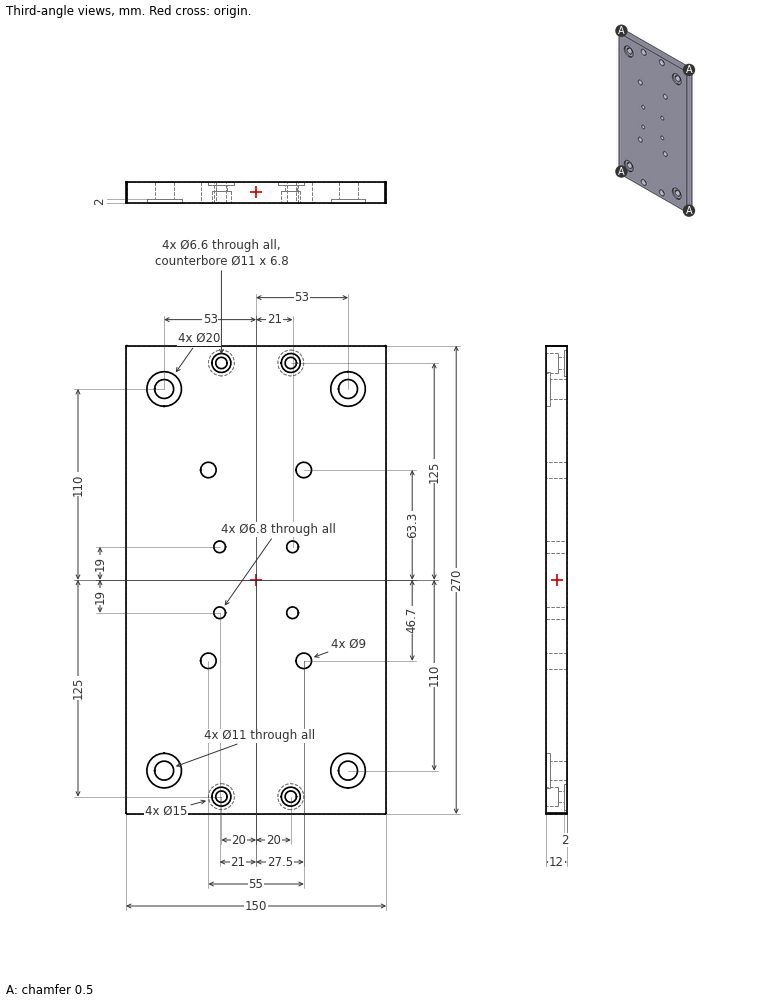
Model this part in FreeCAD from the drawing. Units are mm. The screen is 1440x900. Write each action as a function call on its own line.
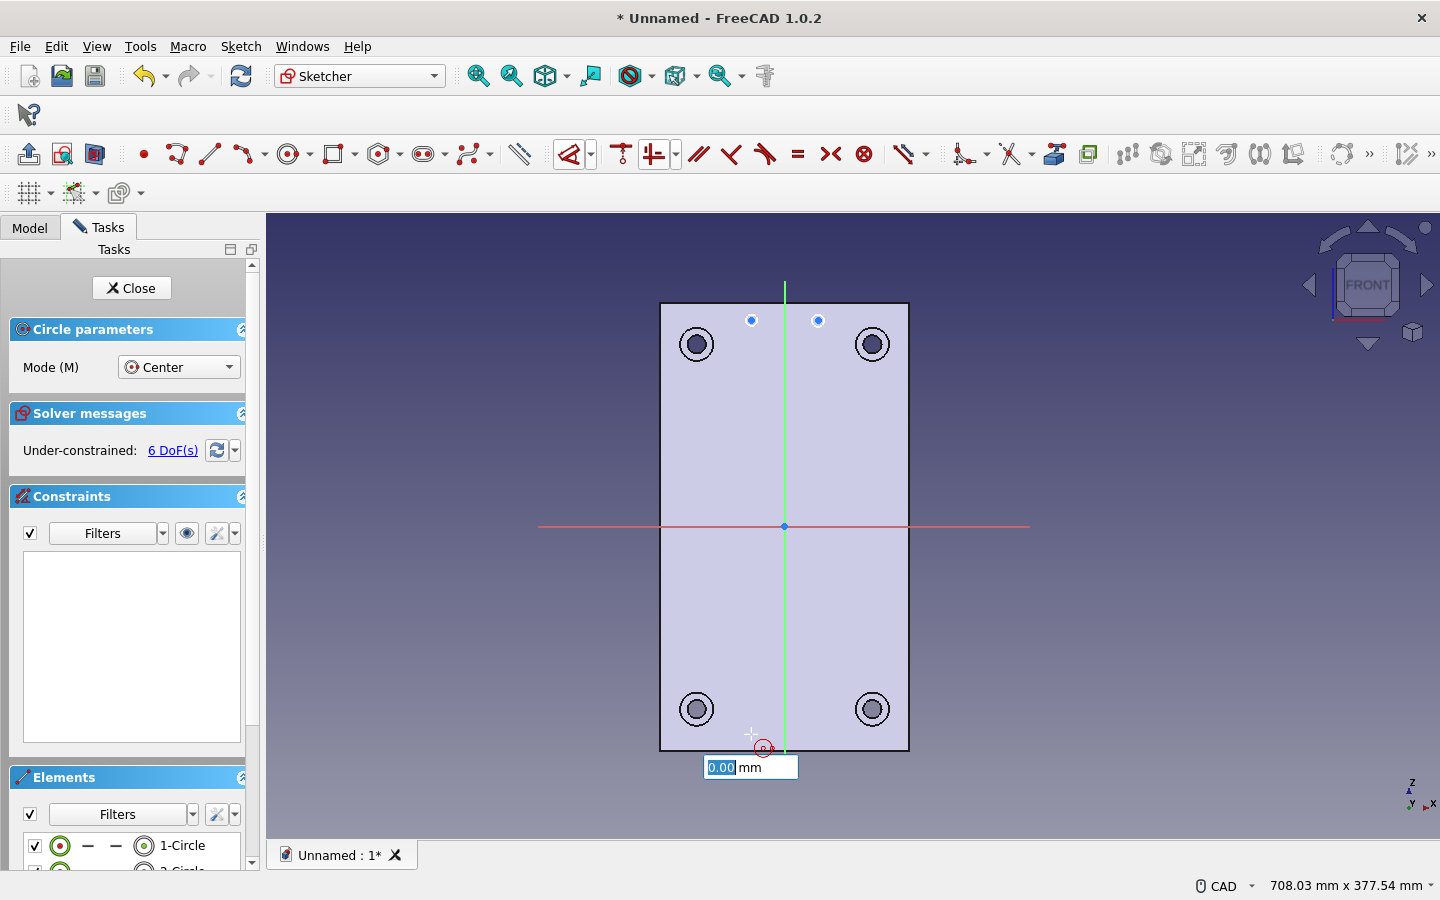
scroll(755, 730, up, 6)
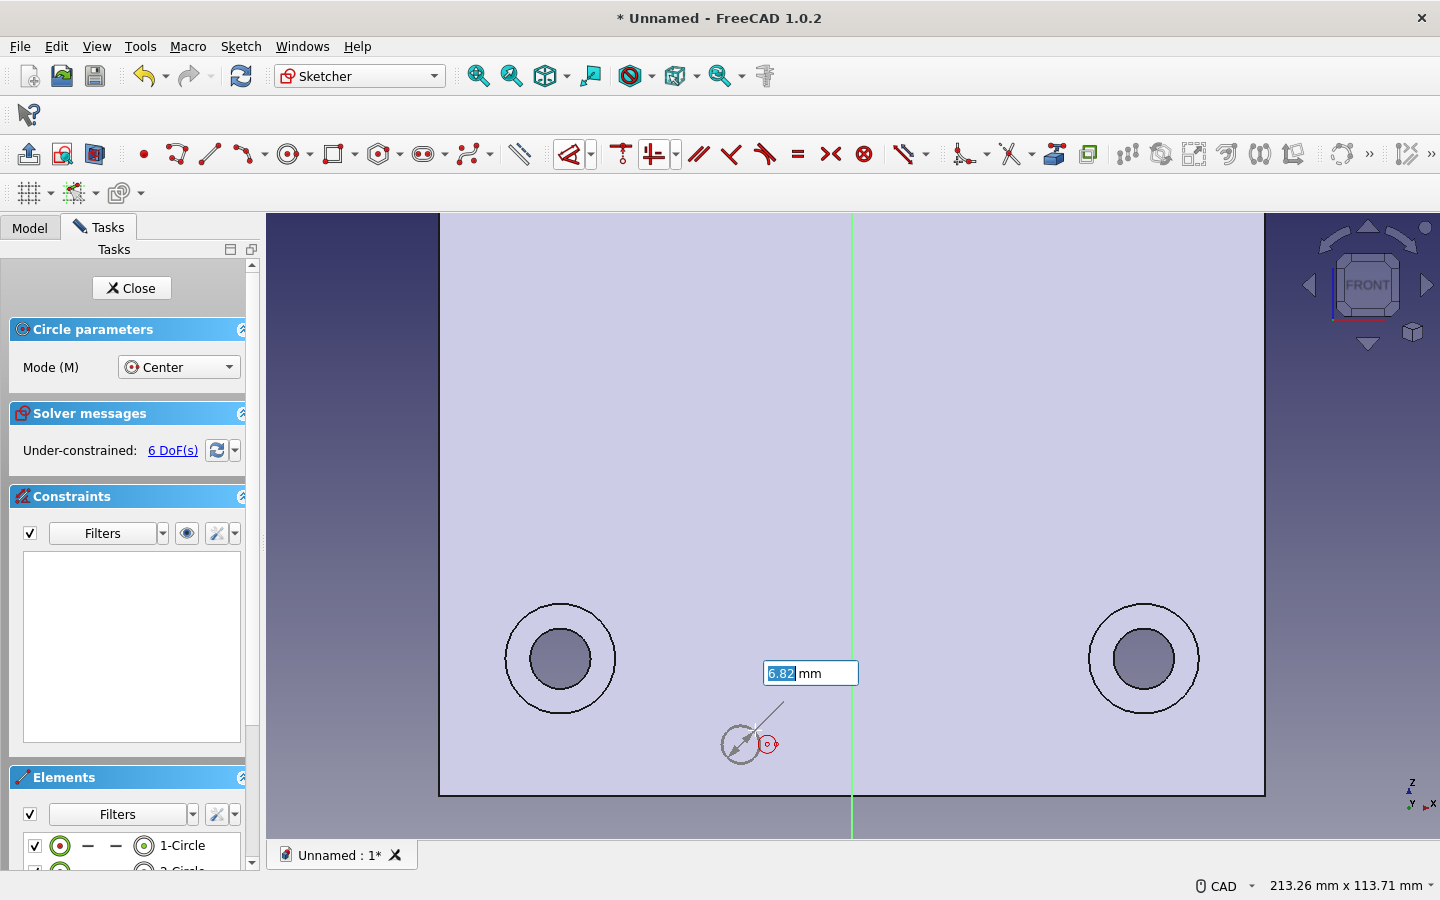
click(755, 728)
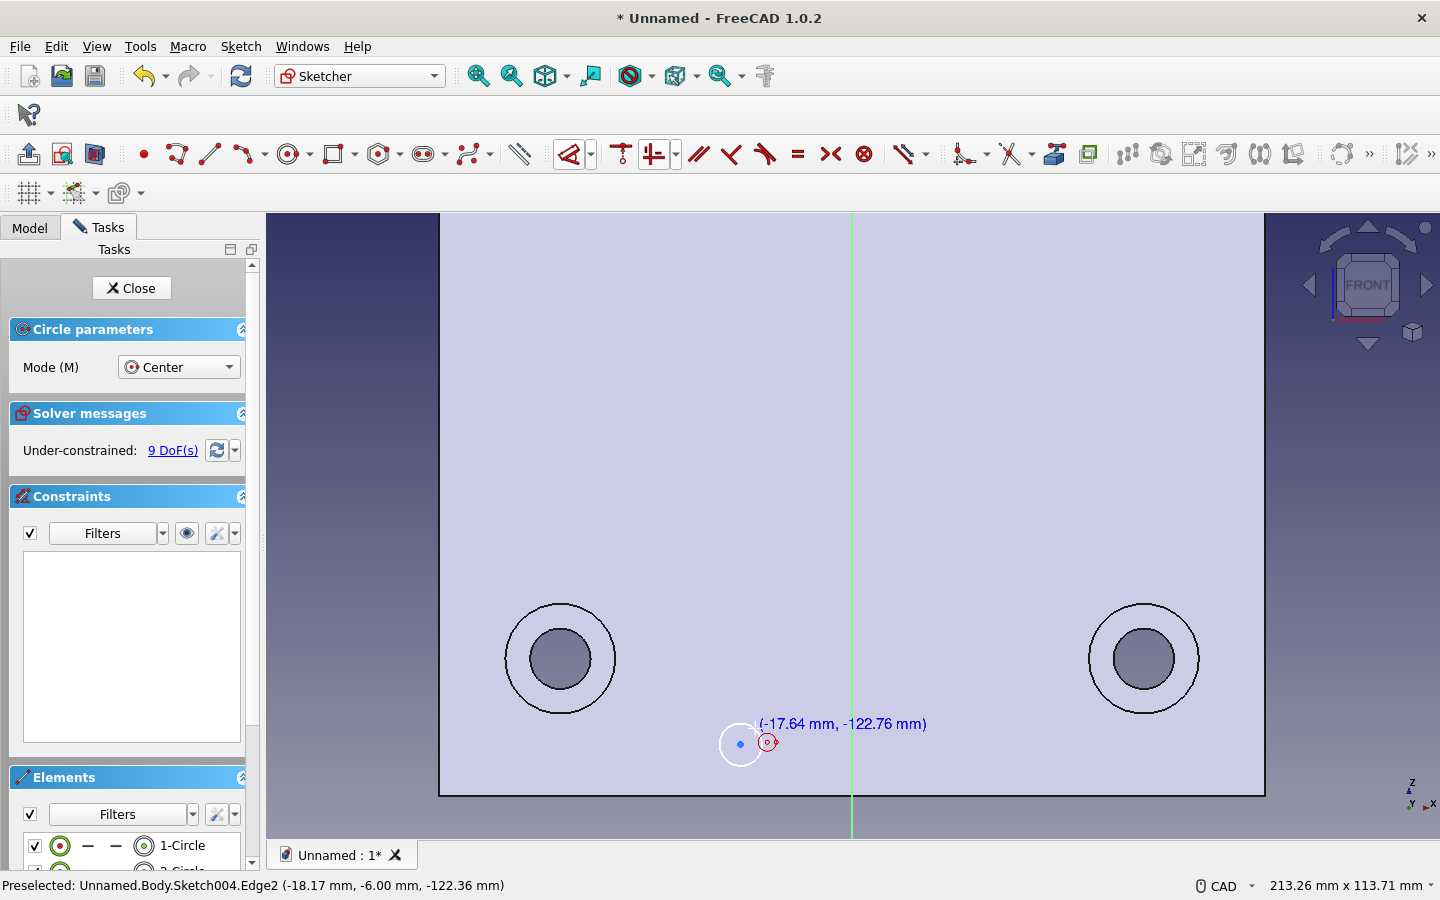
scroll(962, 741, up, 2)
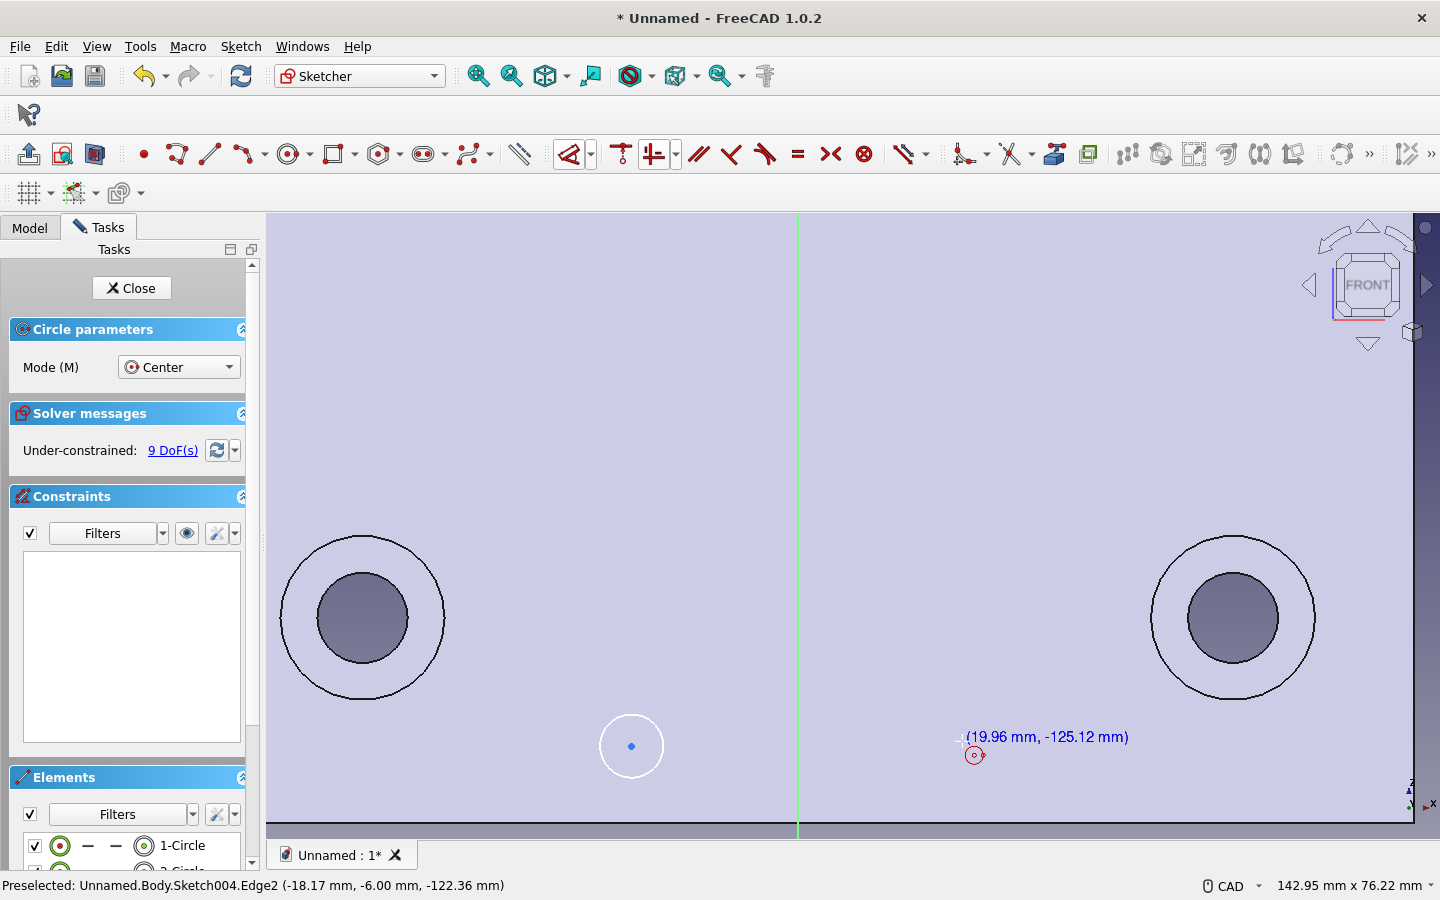
scroll(781, 731, down, 8)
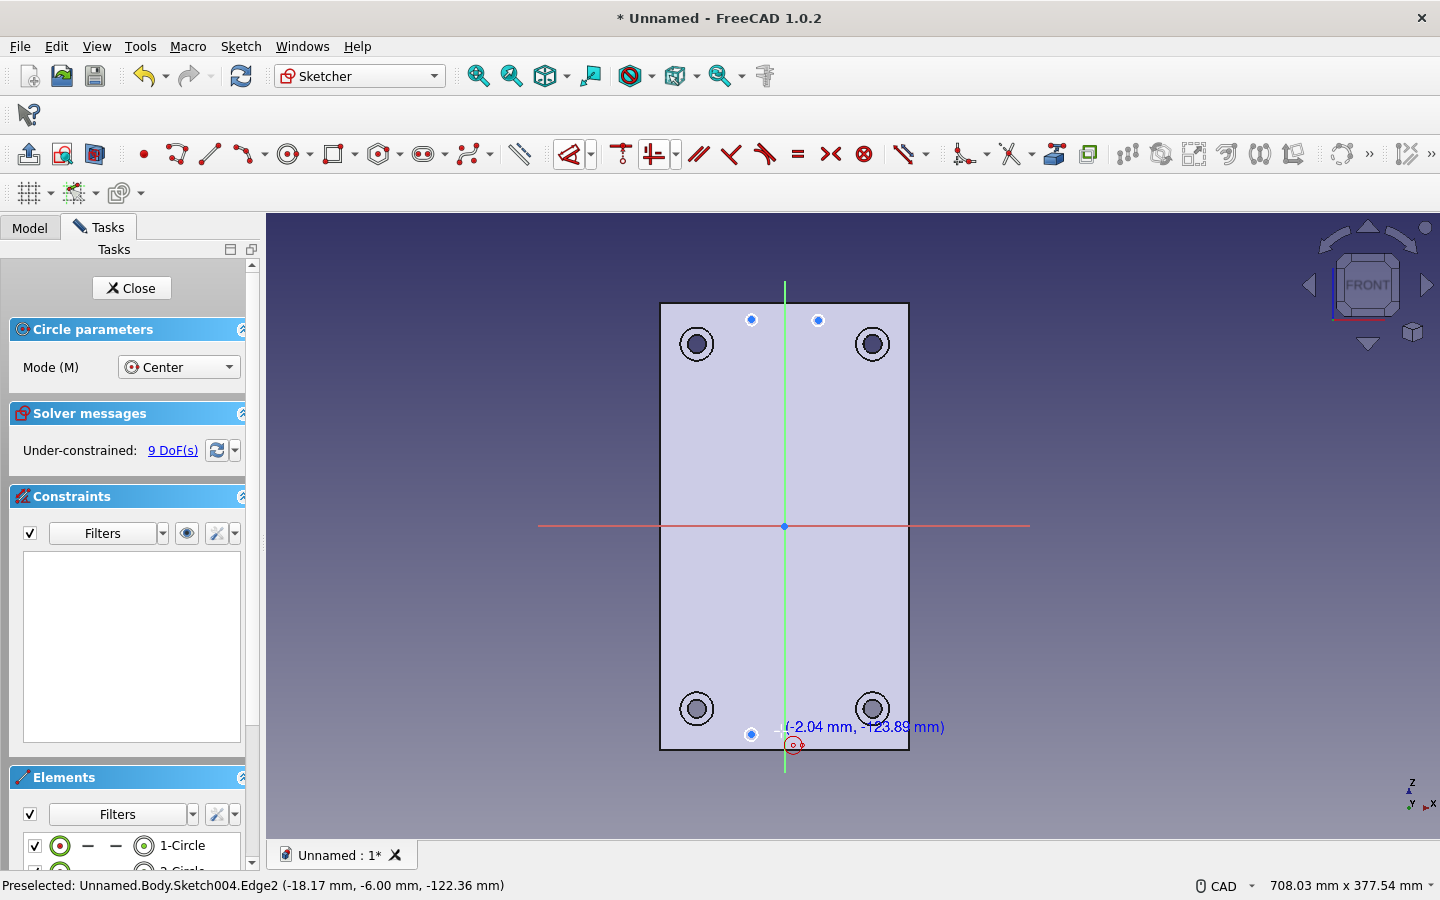
click(818, 734)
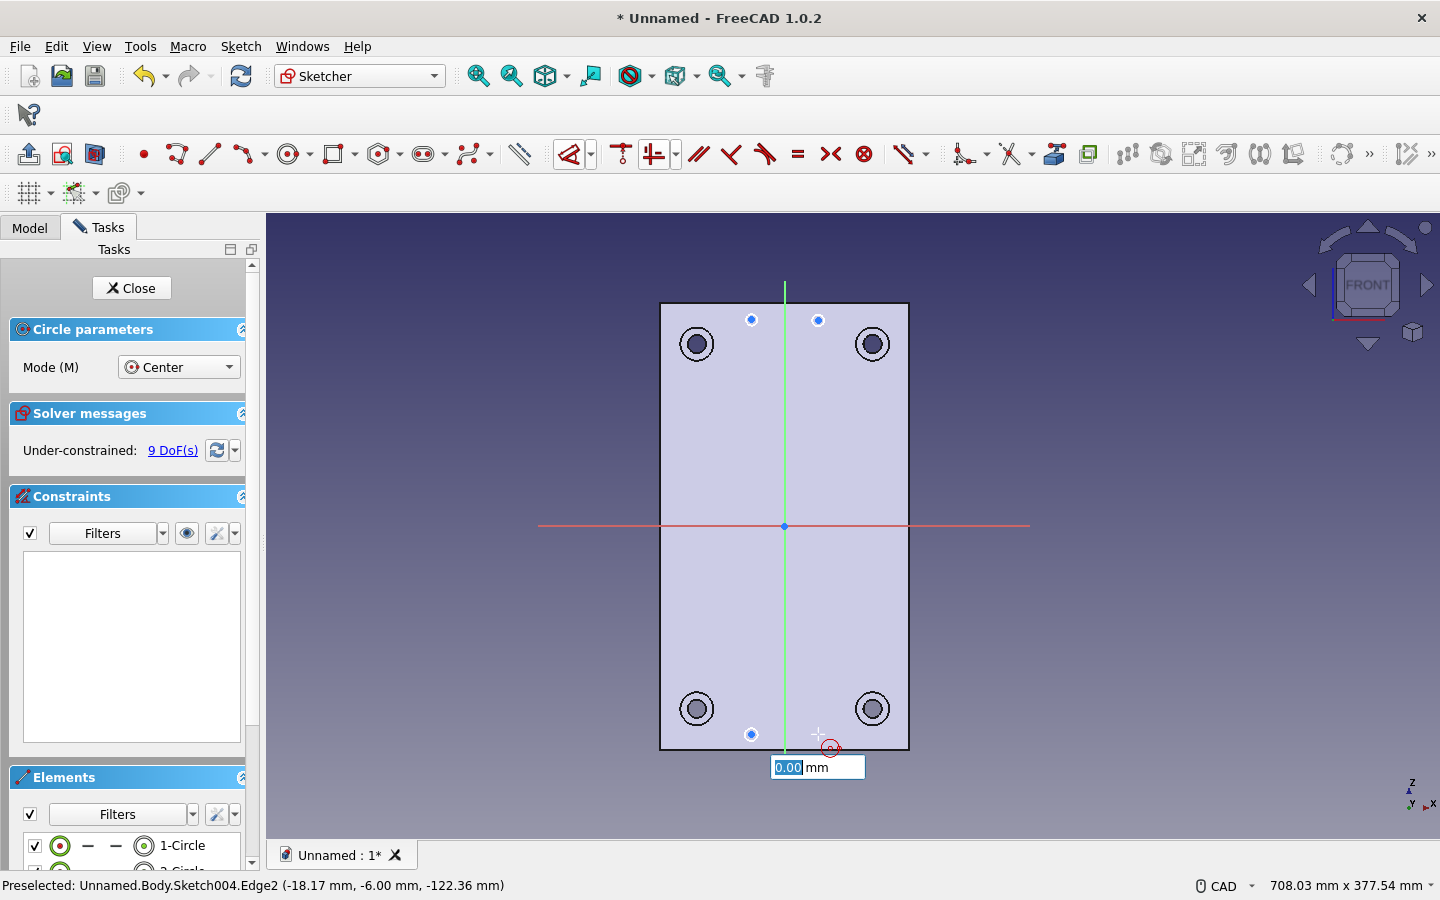
scroll(822, 730, up, 6)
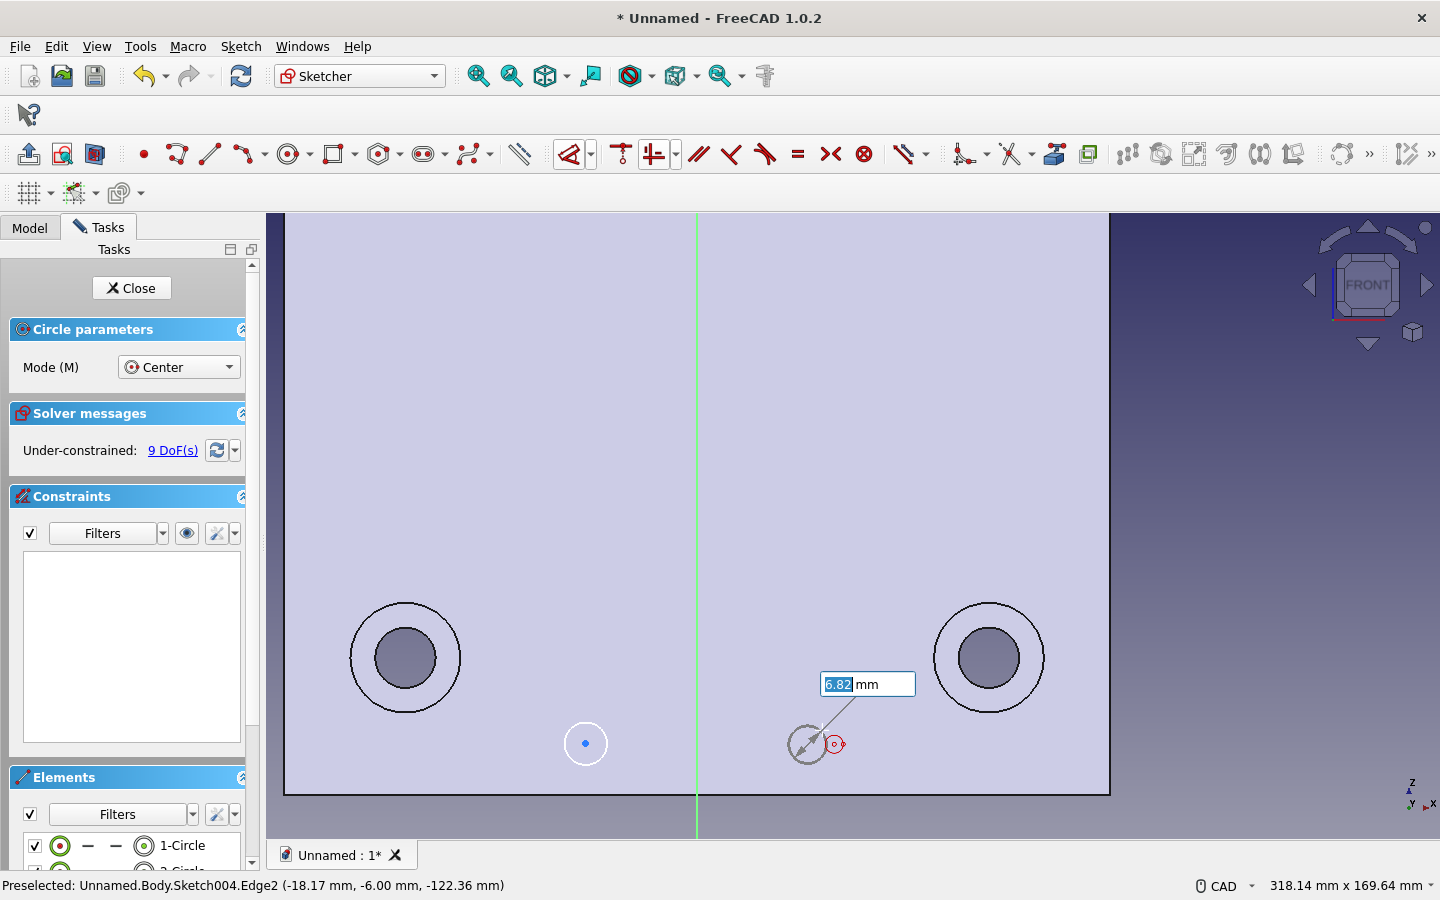
click(820, 728)
key(Escape)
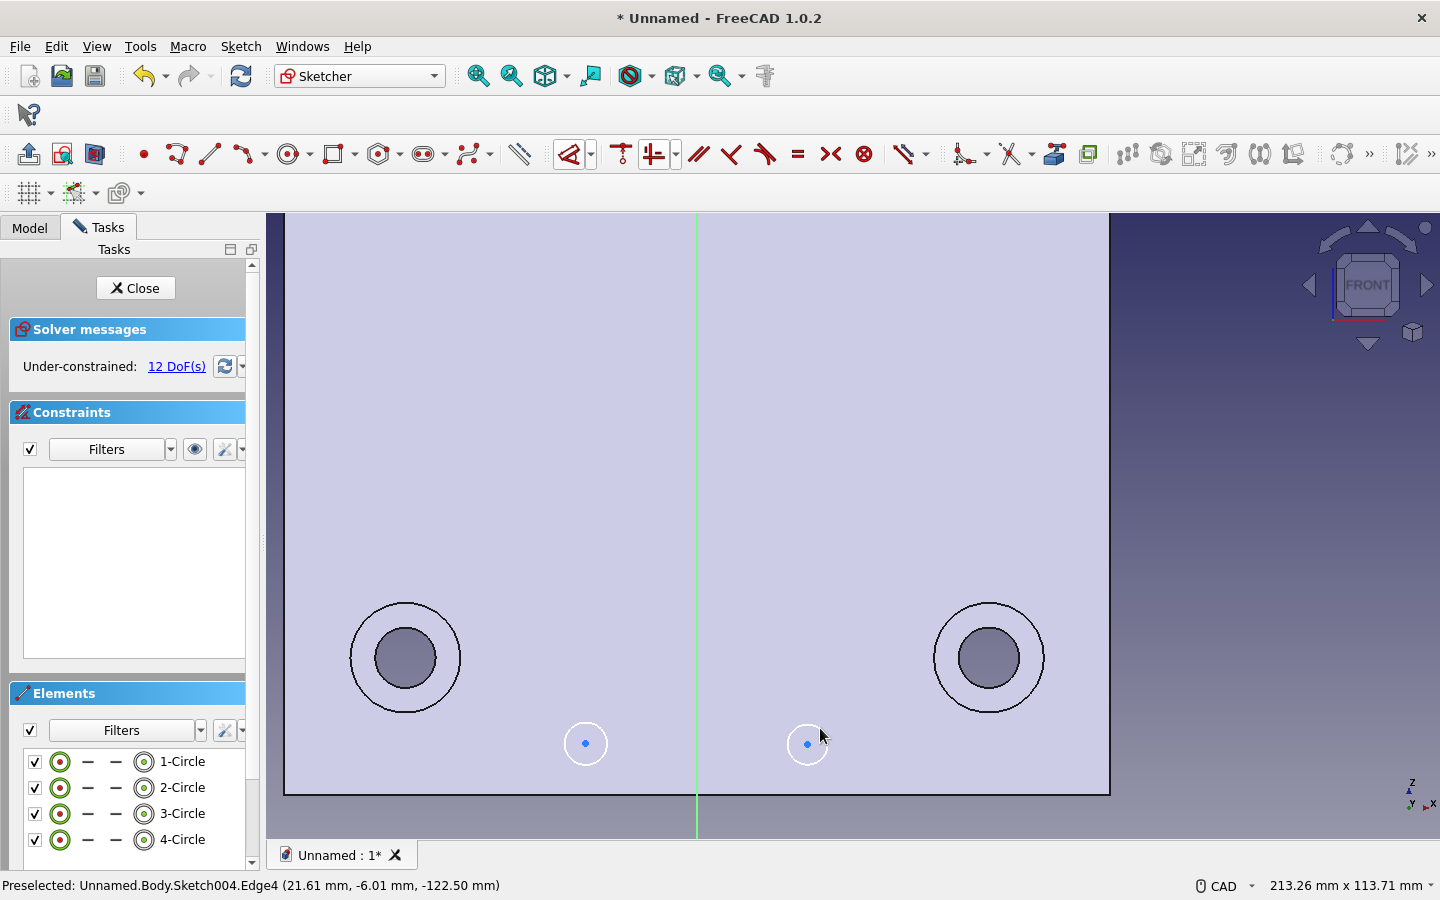
scroll(822, 730, down, 6)